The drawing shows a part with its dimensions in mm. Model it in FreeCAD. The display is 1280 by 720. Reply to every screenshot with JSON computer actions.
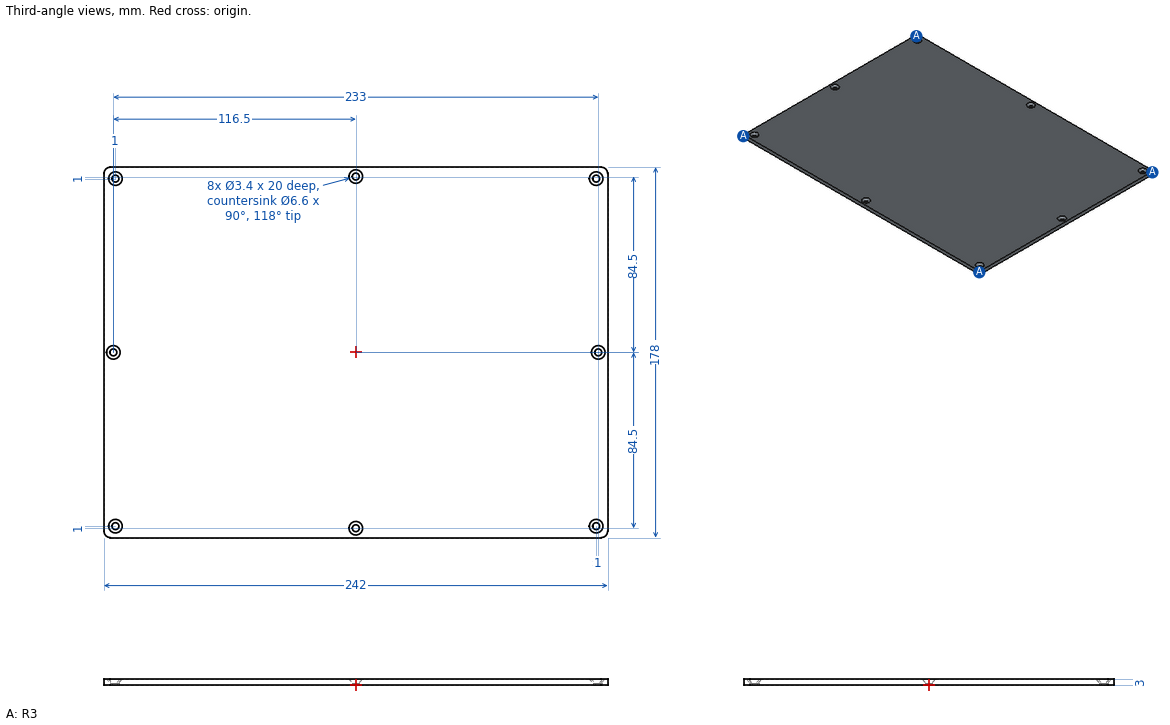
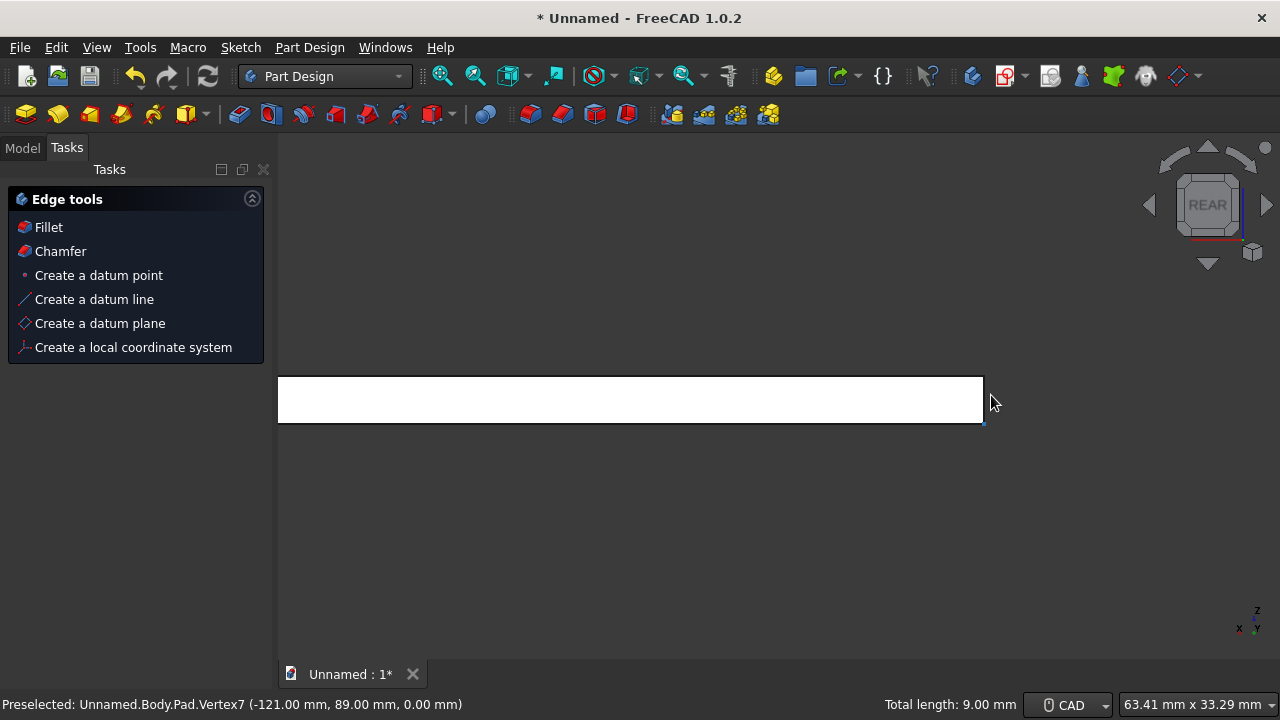
{"action": "left_click", "coordinate": [984, 399], "text": "ctrl"}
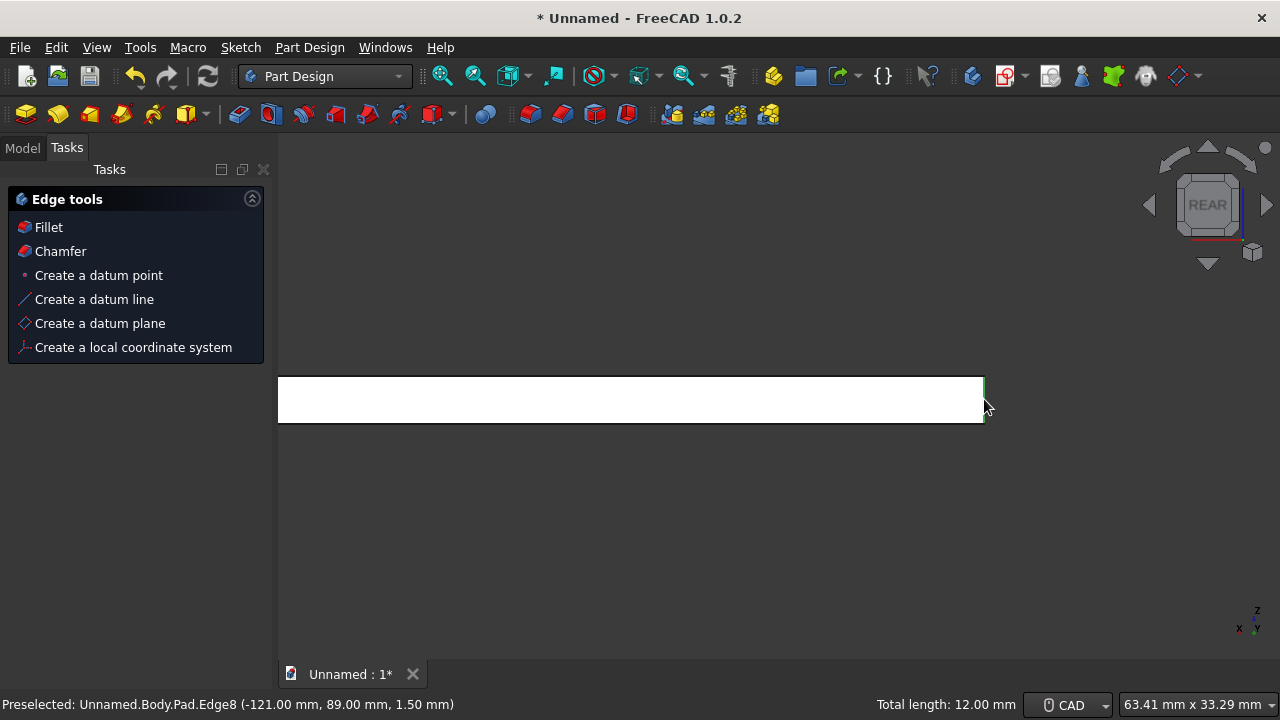
{"action": "left_click", "coordinate": [532, 114]}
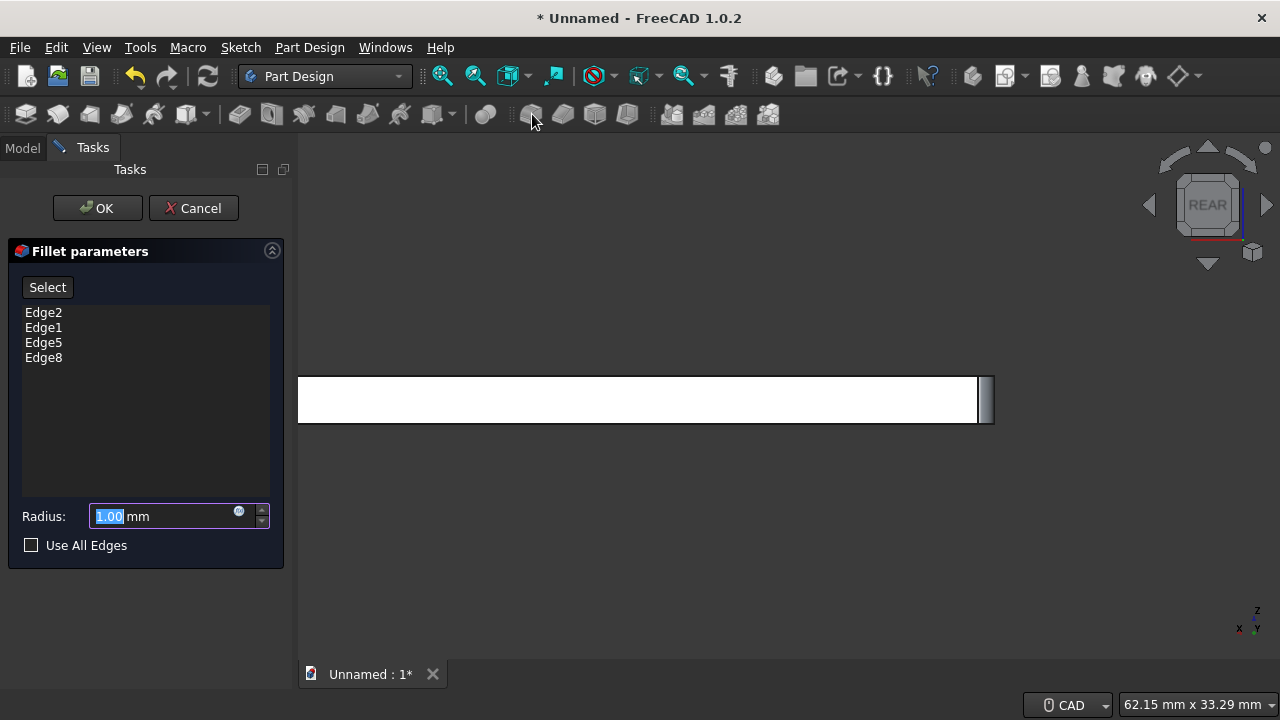
{"action": "type", "text": "3"}
{"action": "key", "text": "Tab"}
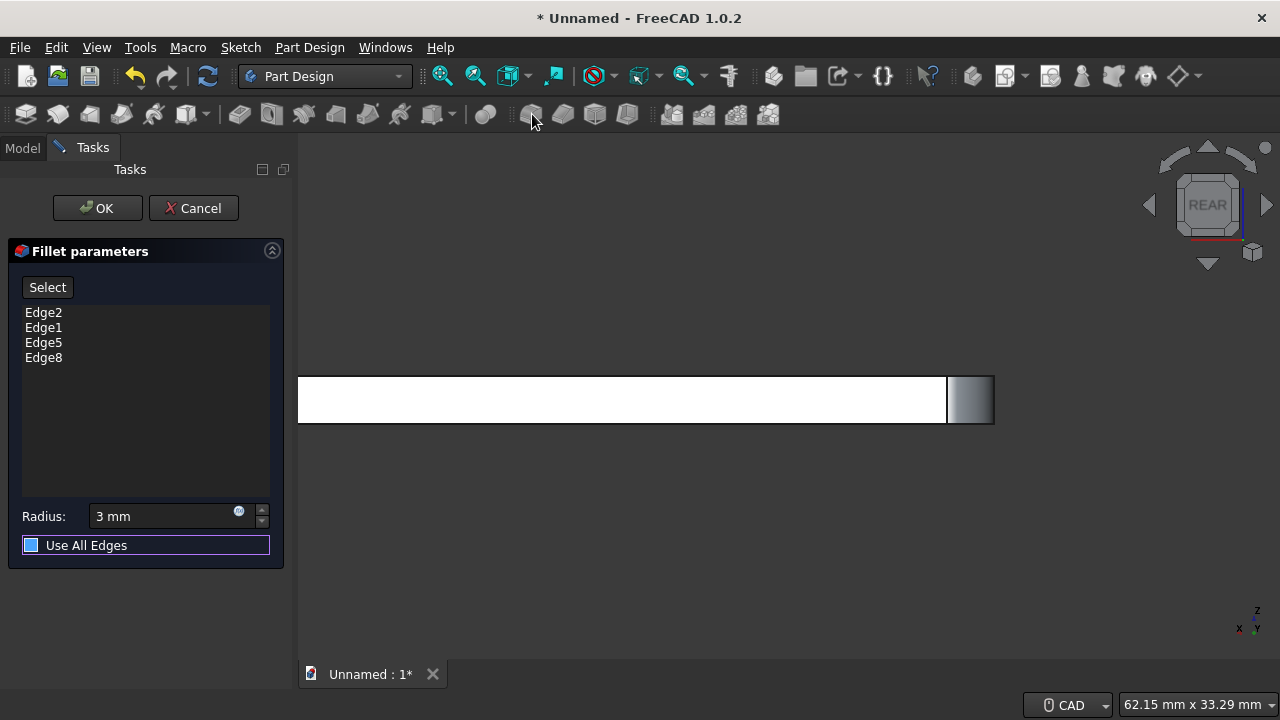
{"action": "left_click", "coordinate": [98, 208]}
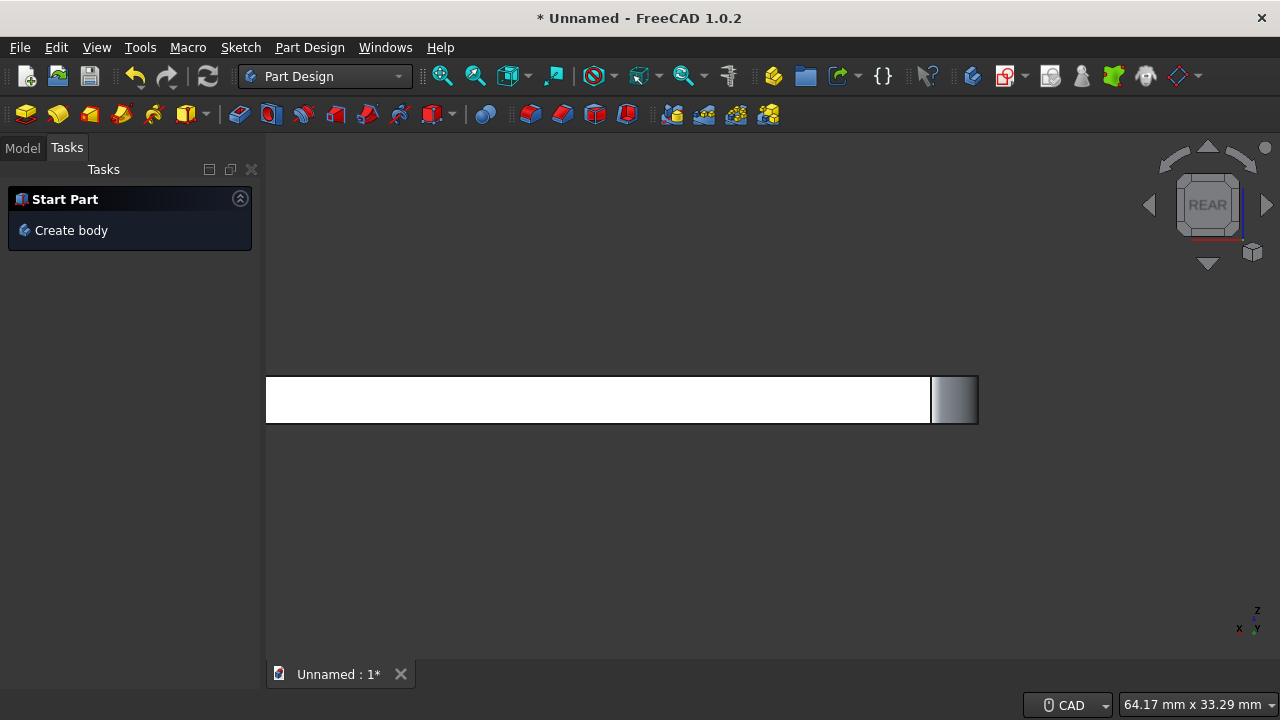
{"action": "left_click", "coordinate": [444, 76]}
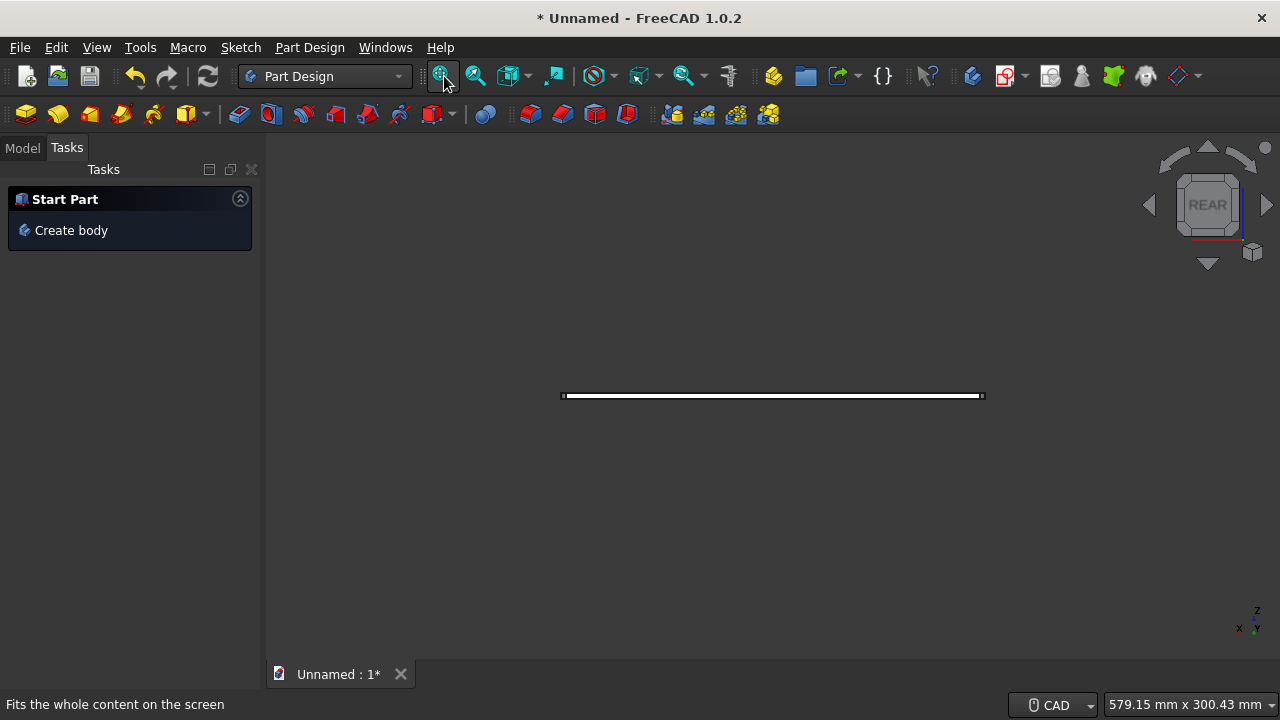
{"action": "key", "text": "0"}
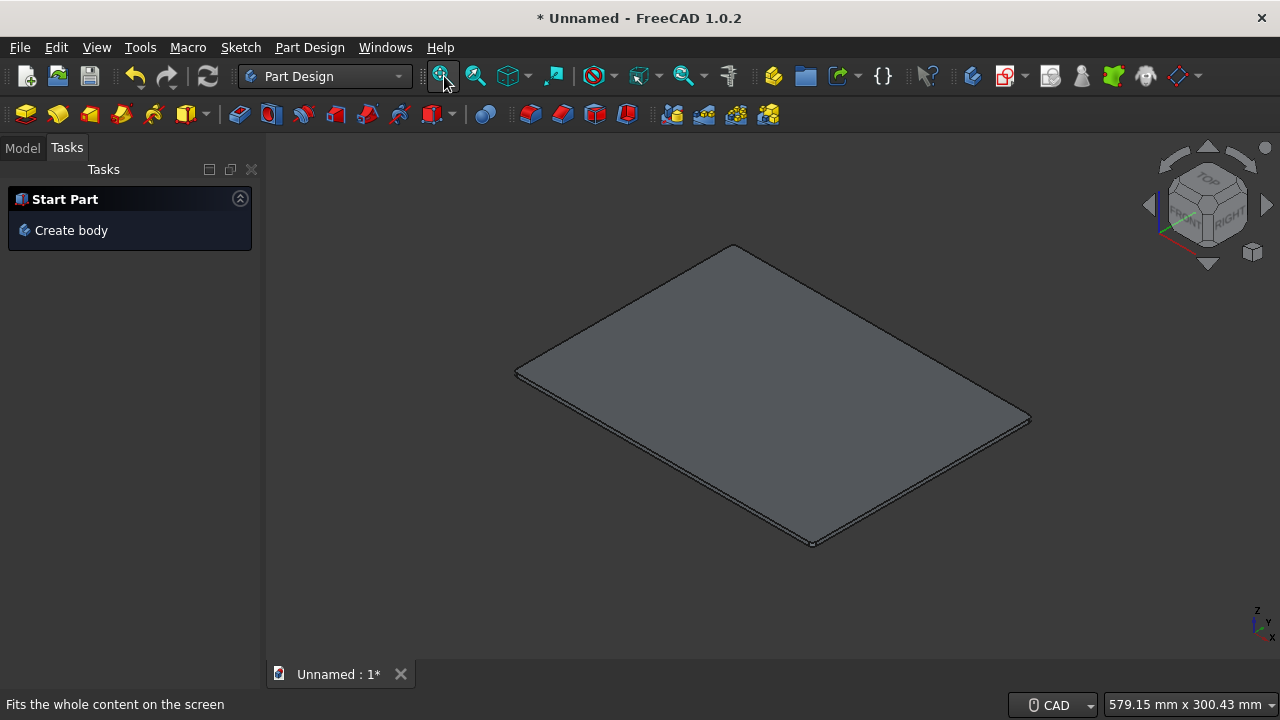
{"action": "left_click", "coordinate": [773, 393]}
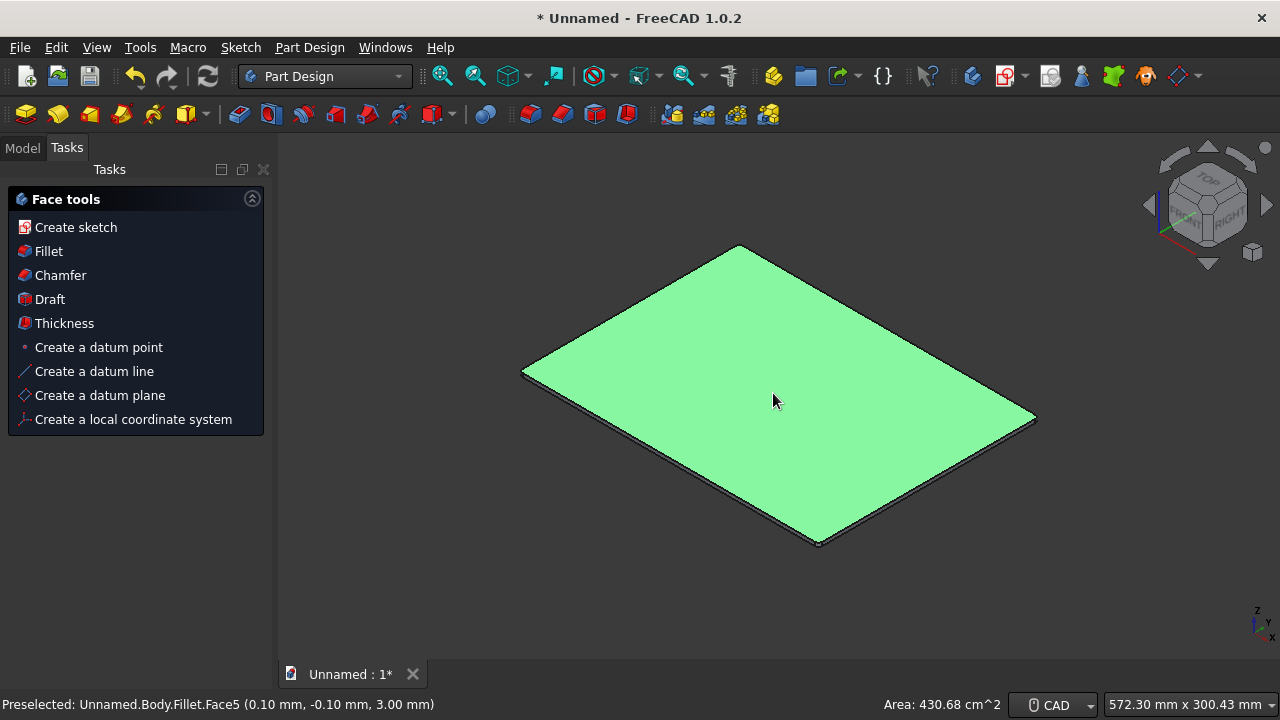
{"action": "left_click", "coordinate": [1006, 76]}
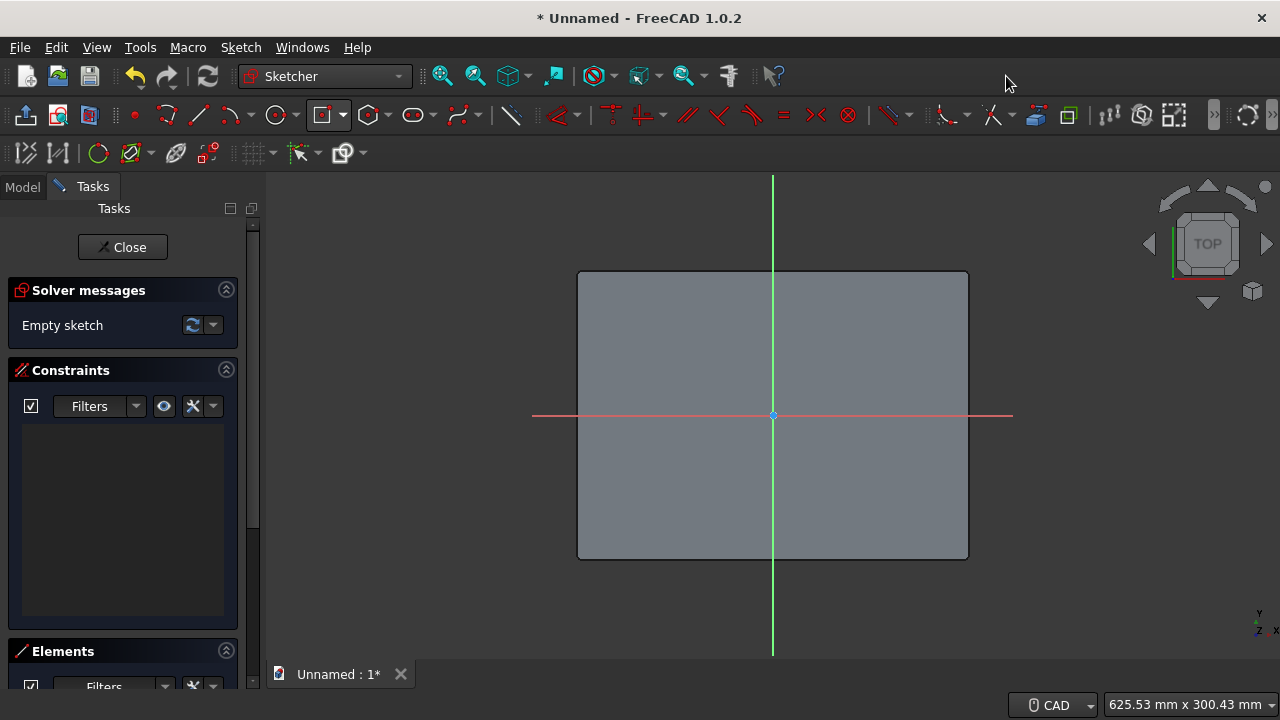
{"action": "left_click", "coordinate": [276, 116]}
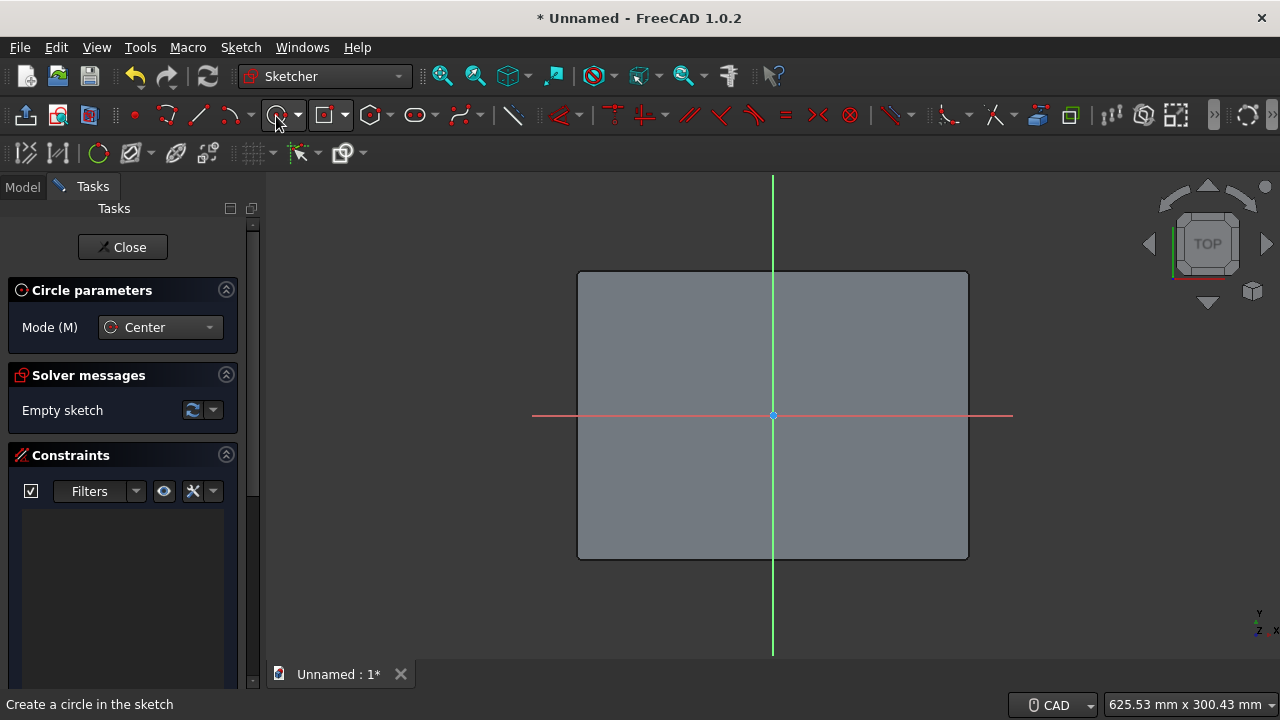
{"action": "scroll", "coordinate": [773, 279], "scroll_direction": "up", "scroll_amount": 11}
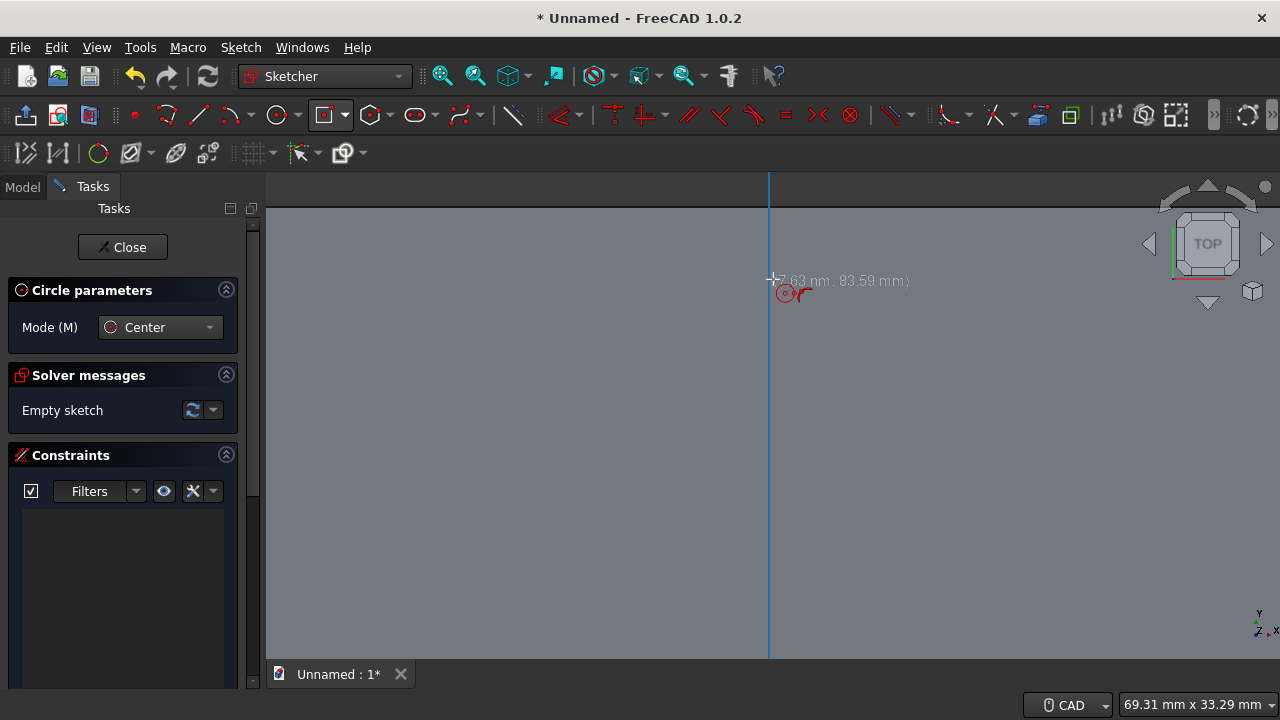
{"action": "scroll", "coordinate": [696, 279], "scroll_direction": "down", "scroll_amount": 11}